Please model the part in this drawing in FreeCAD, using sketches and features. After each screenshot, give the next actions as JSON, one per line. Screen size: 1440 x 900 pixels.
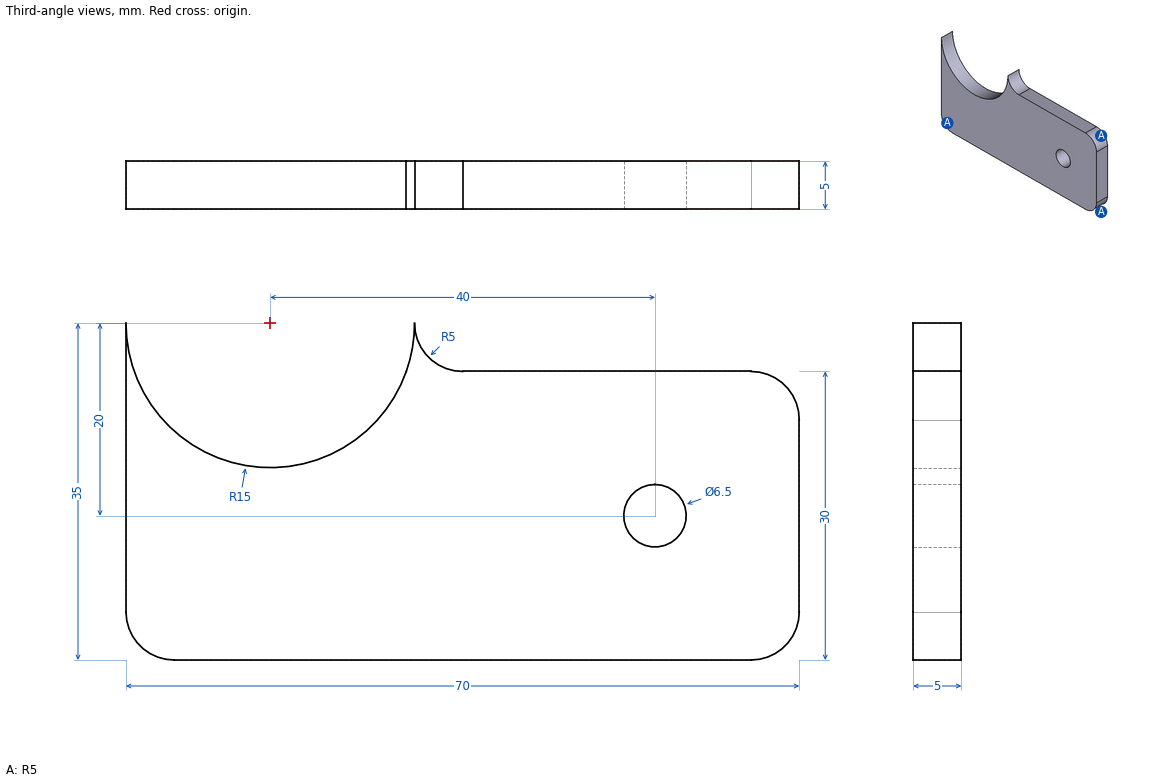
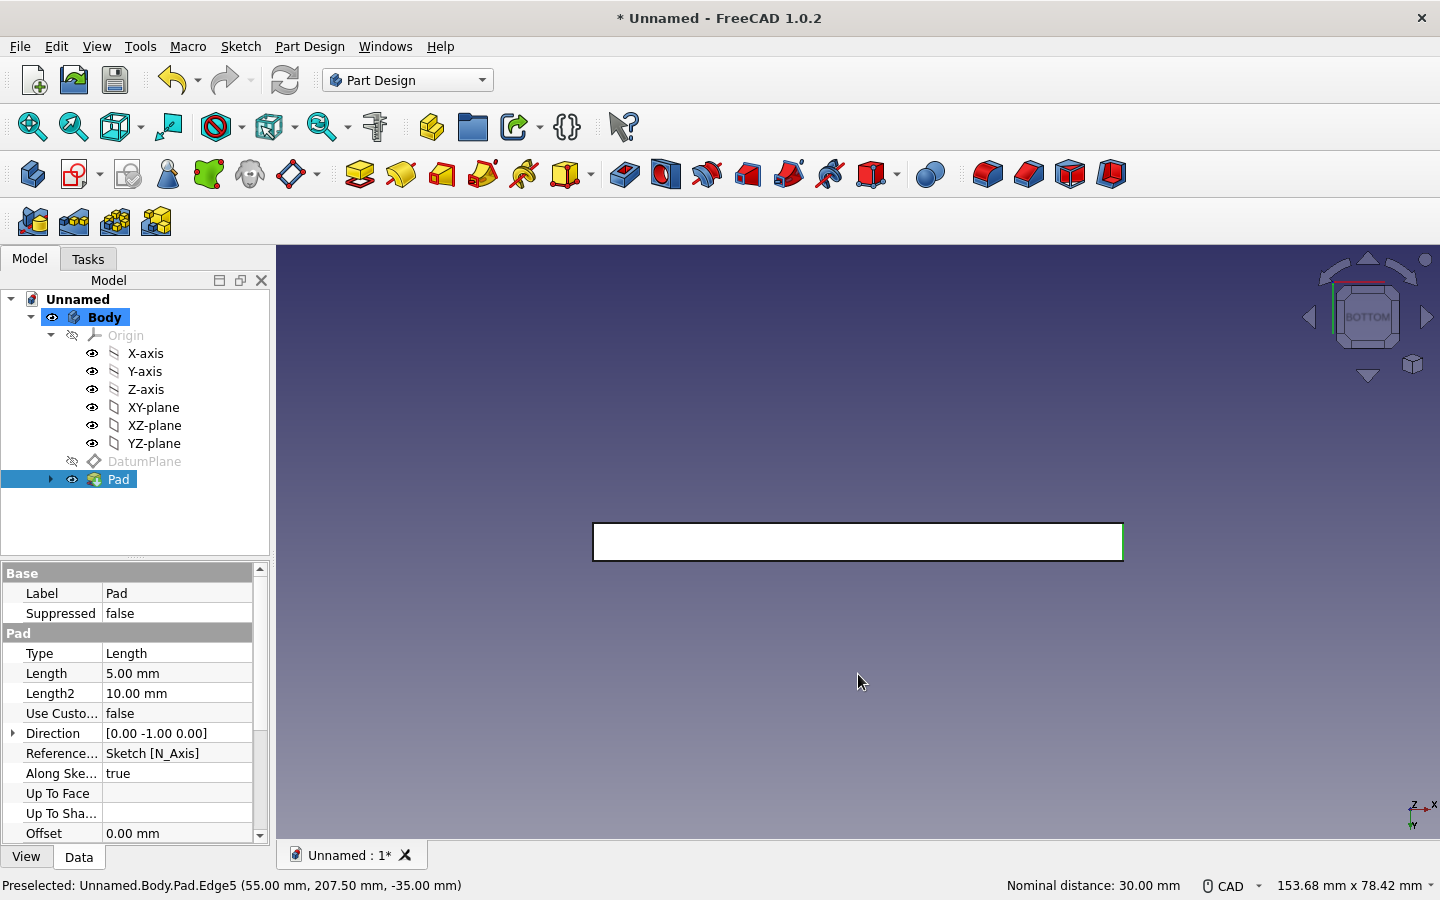
{"action": "left_click", "coordinate": [593, 541], "text": "ctrl"}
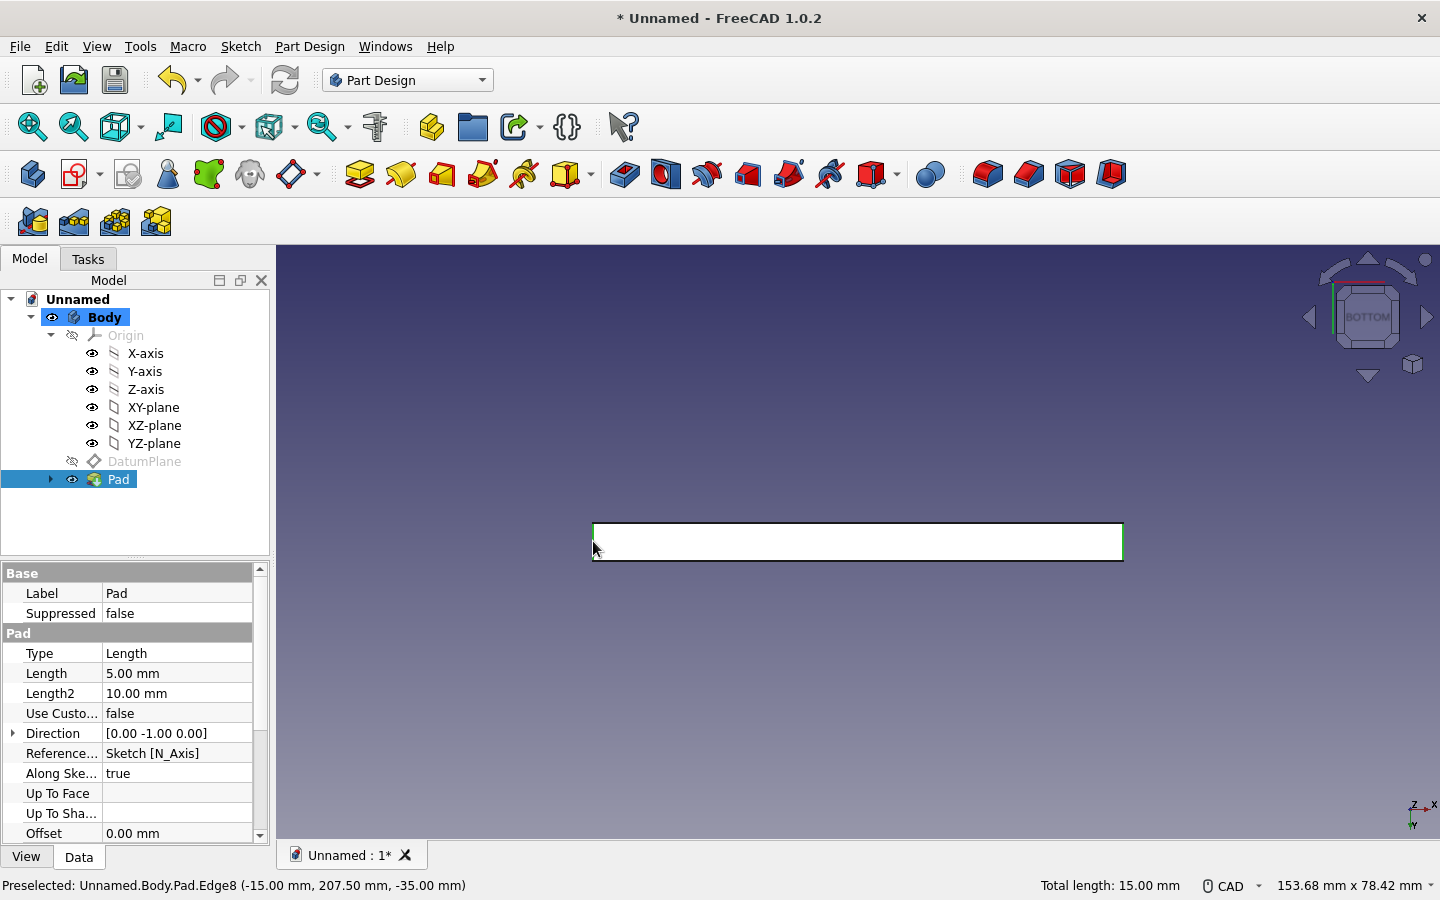
{"action": "left_click", "coordinate": [988, 174]}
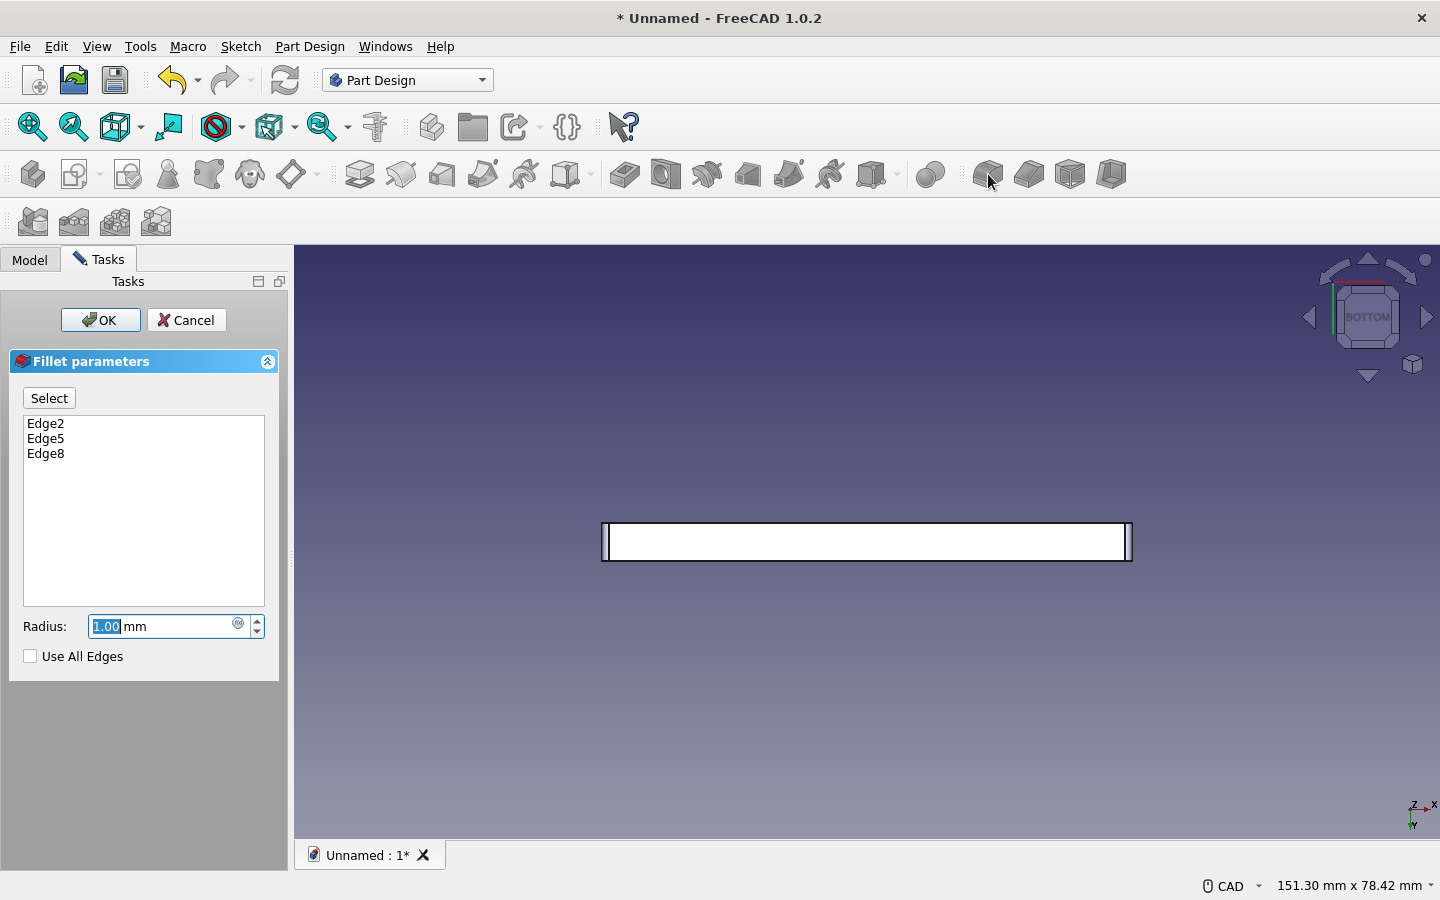
{"action": "type", "text": "5"}
{"action": "key", "text": "Tab"}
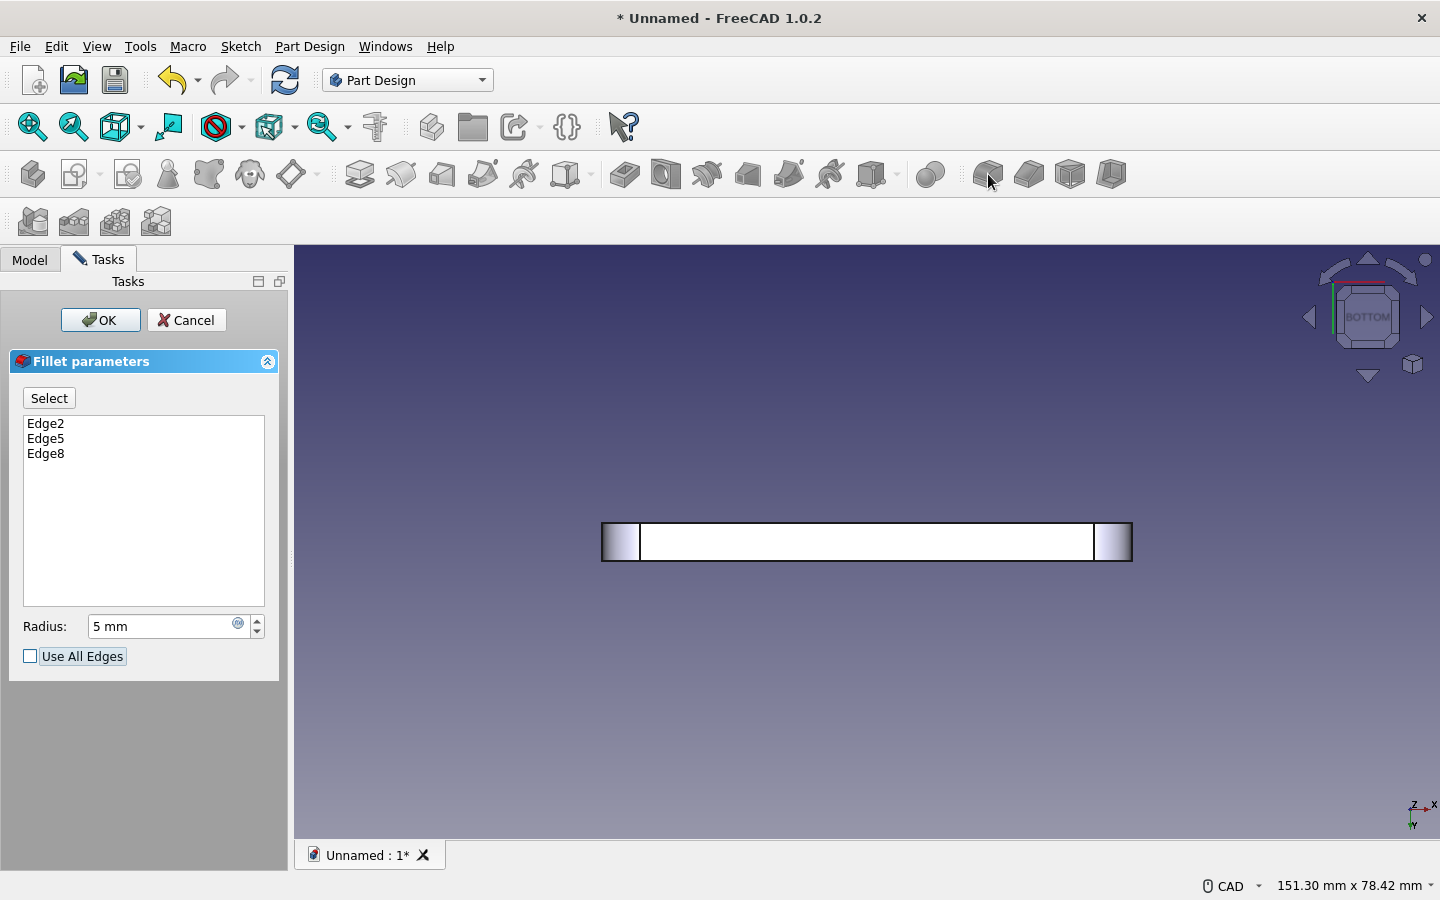
{"action": "left_click", "coordinate": [101, 320]}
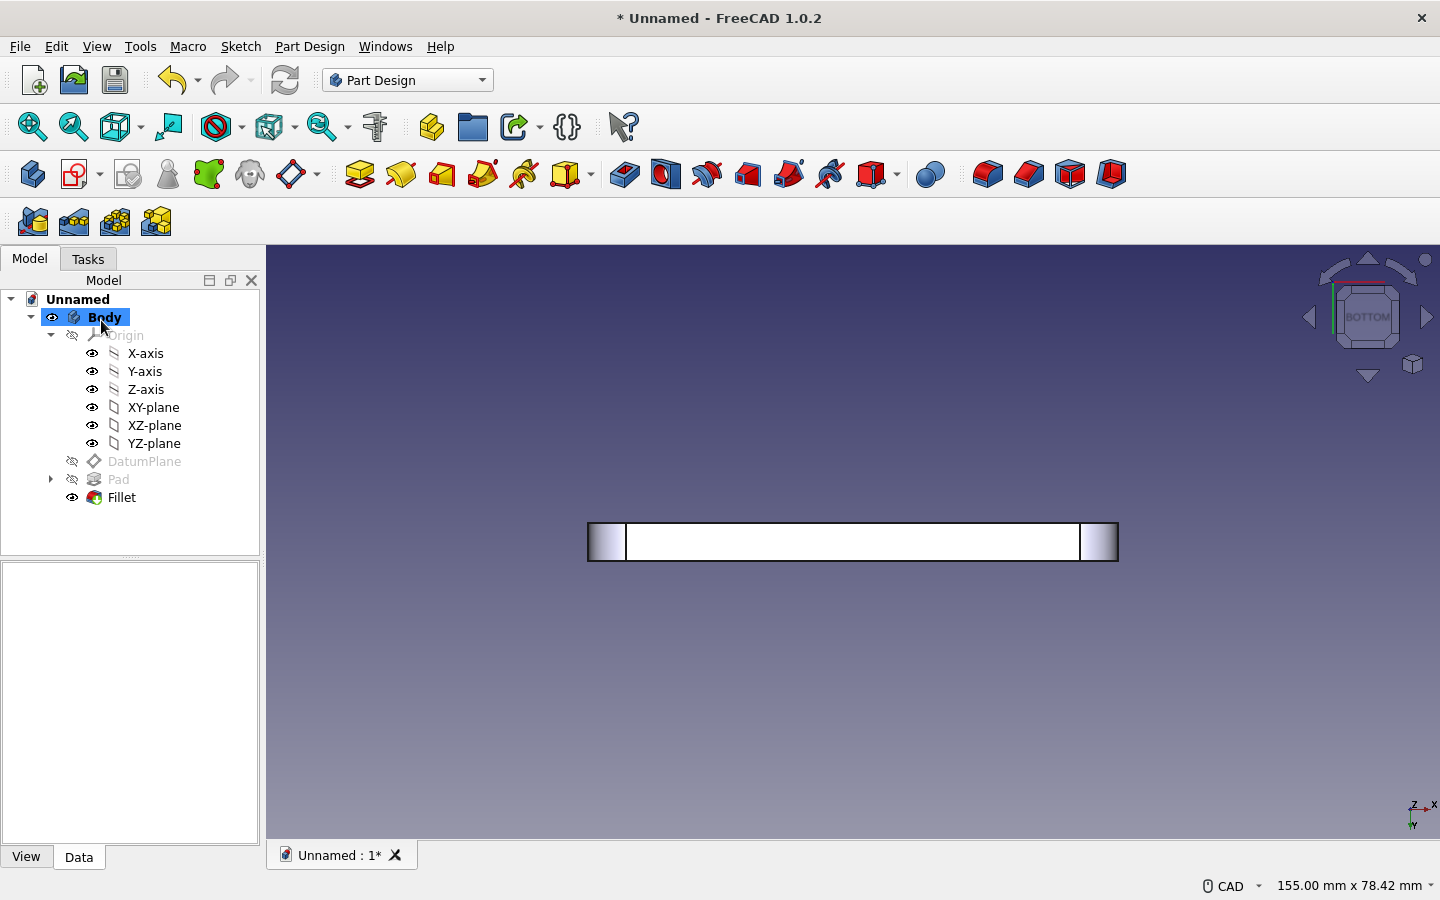
{"action": "key", "text": "4"}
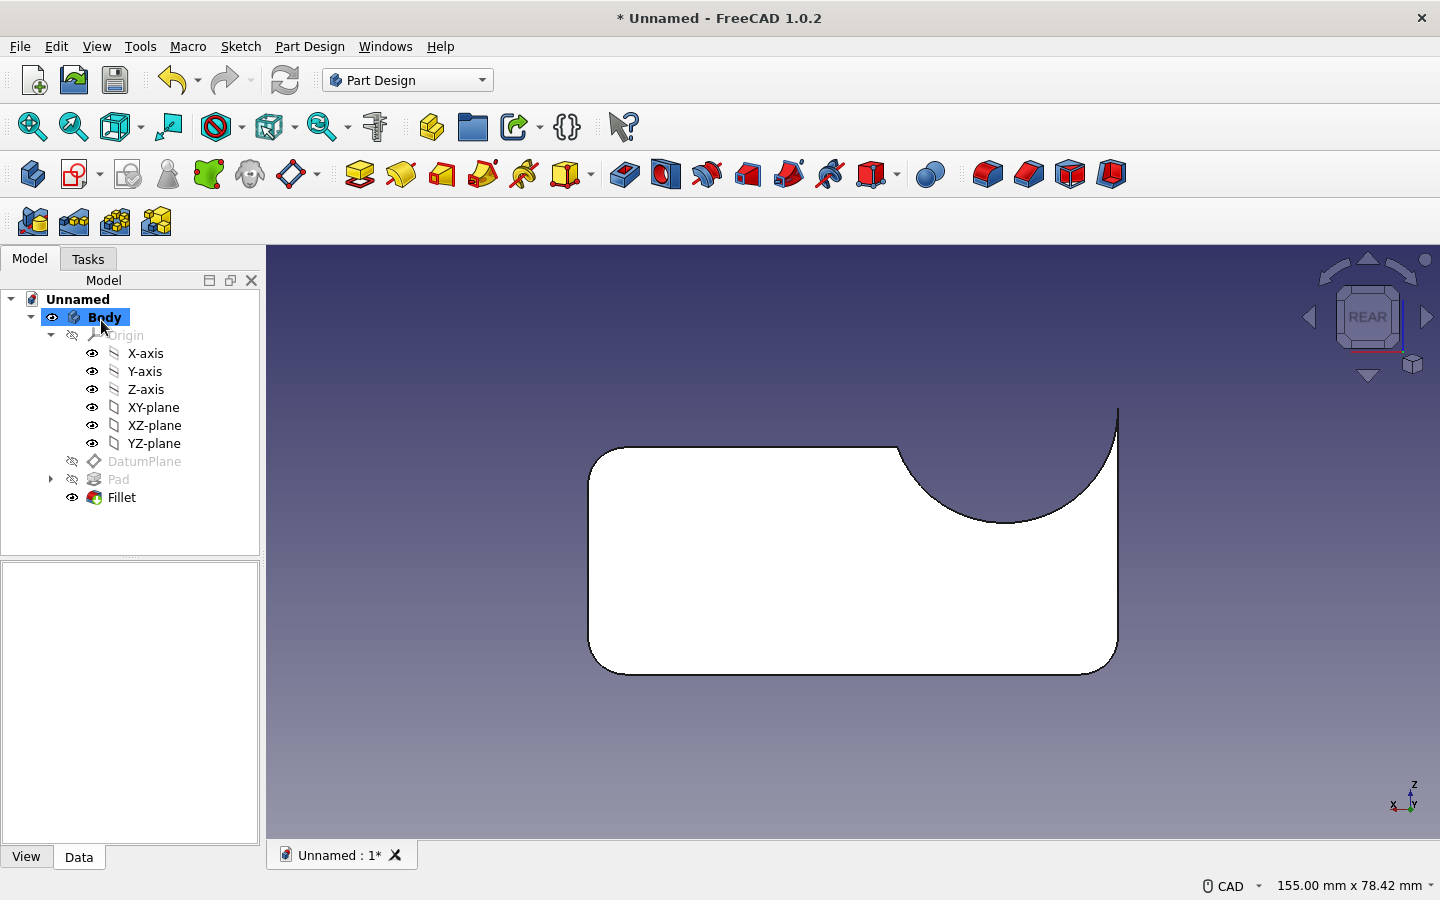
{"action": "left_click", "coordinate": [702, 541]}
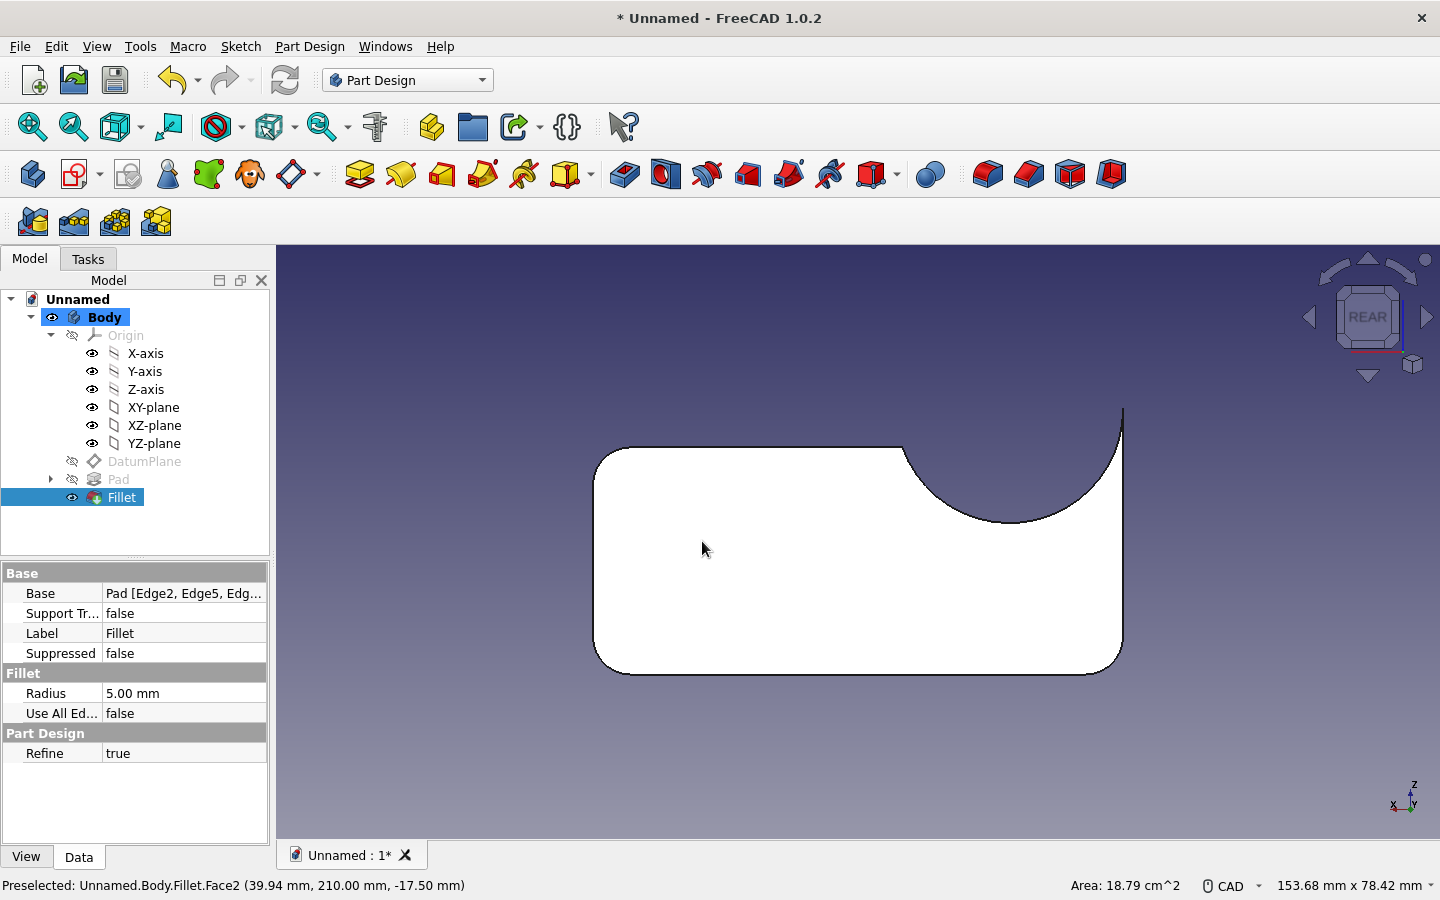
{"action": "left_click", "coordinate": [74, 174]}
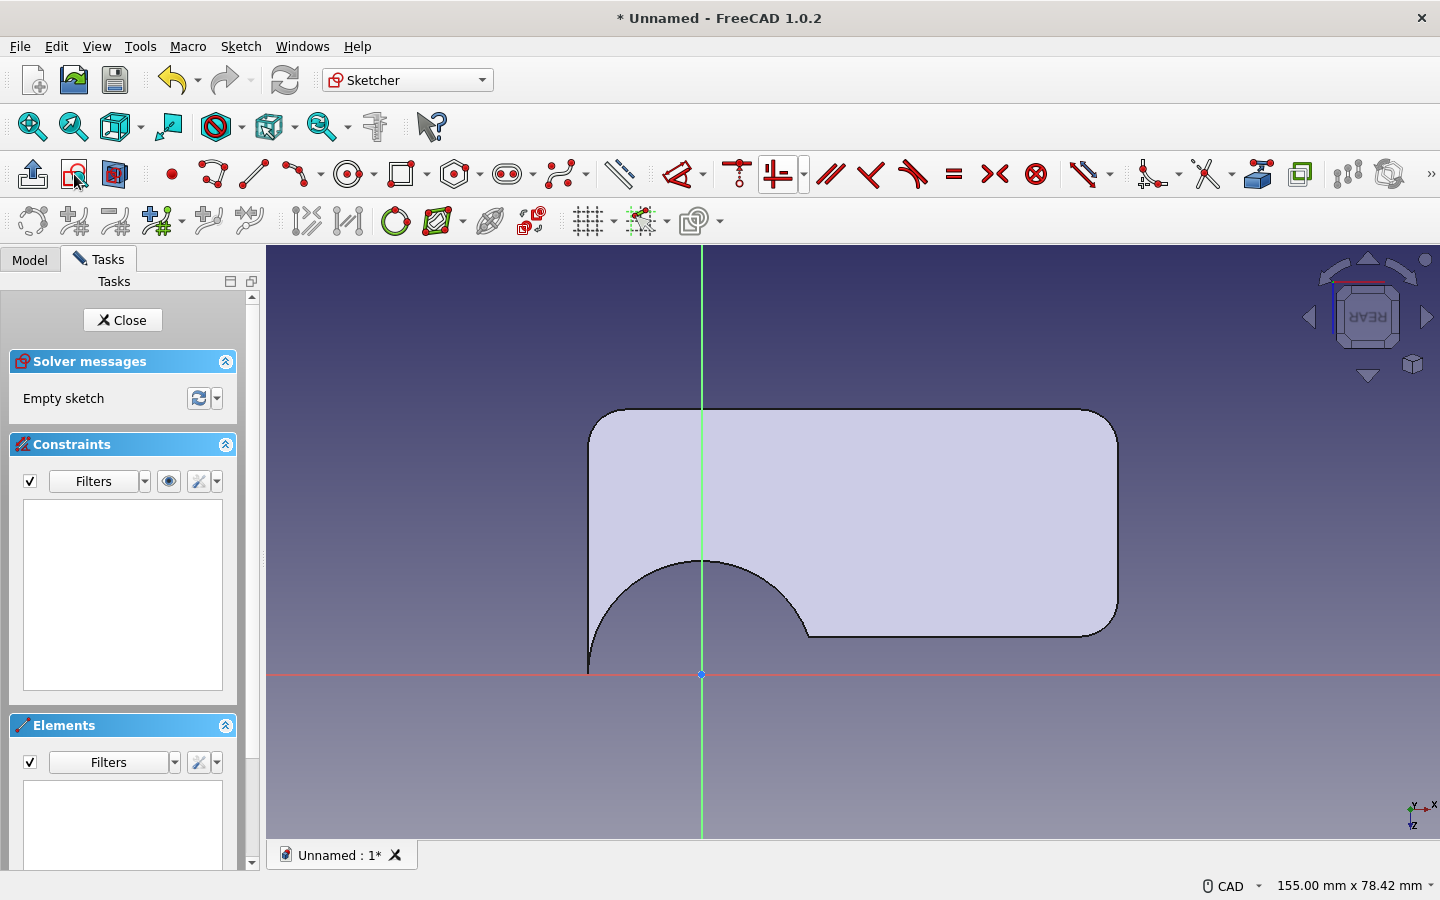
{"action": "scroll", "coordinate": [1039, 520], "scroll_direction": "up", "scroll_amount": 10}